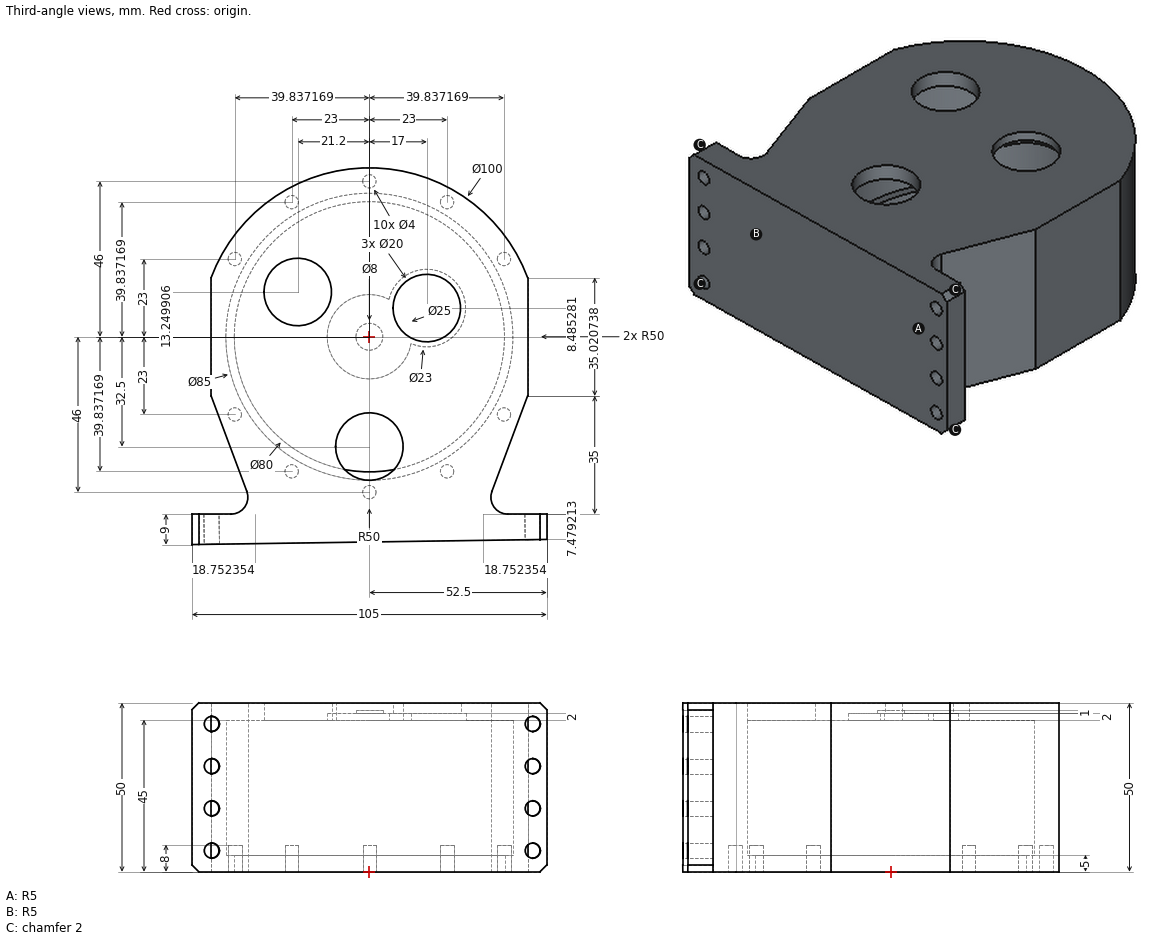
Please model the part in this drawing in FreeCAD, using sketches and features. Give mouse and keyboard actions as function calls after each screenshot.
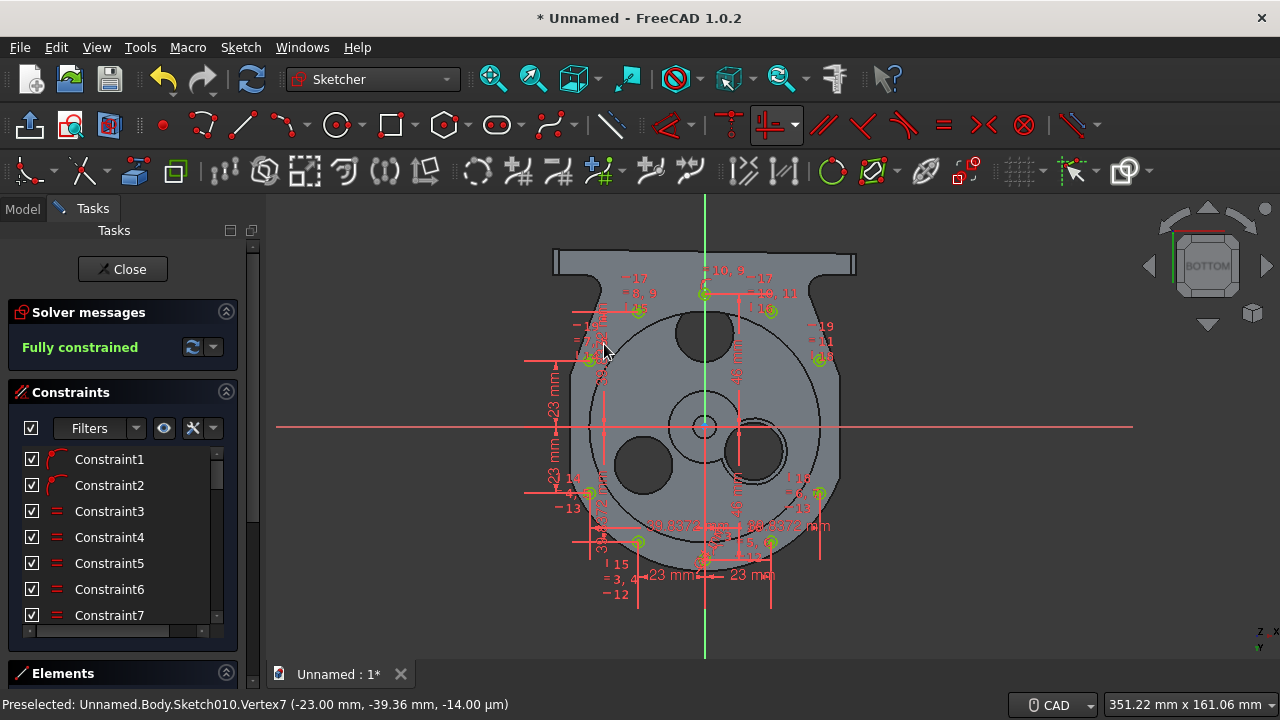
click(123, 269)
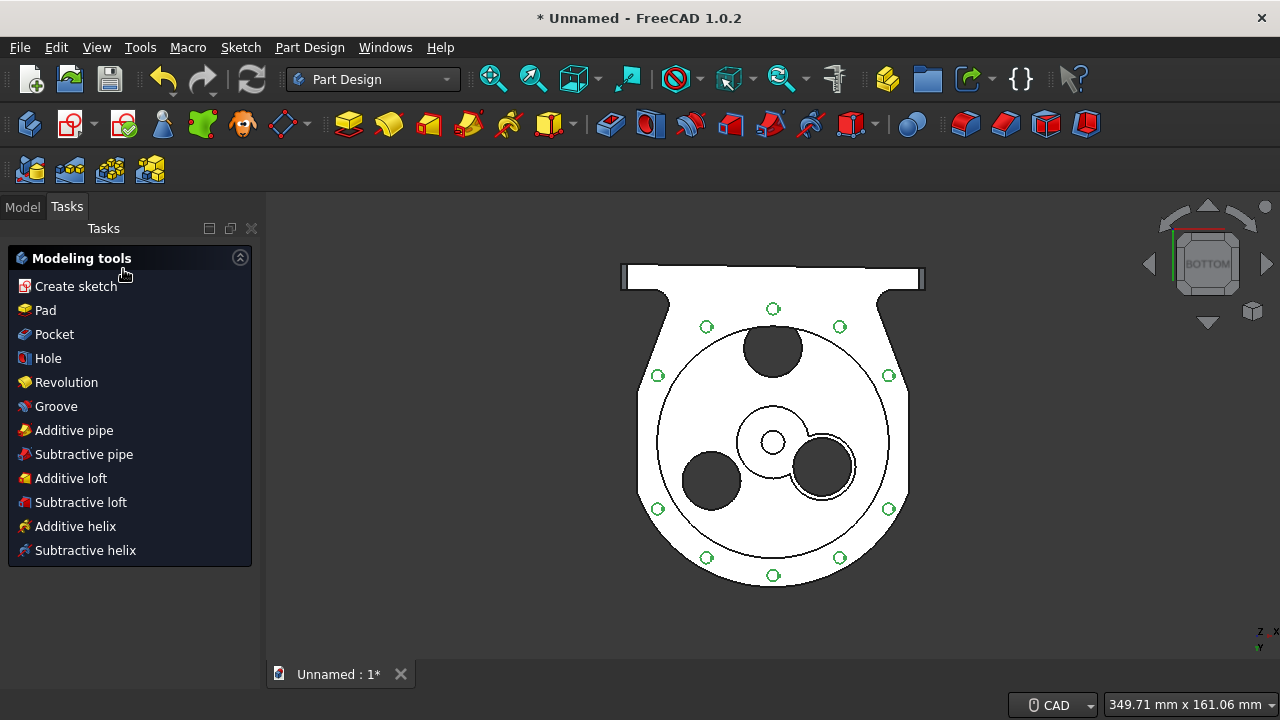
click(612, 124)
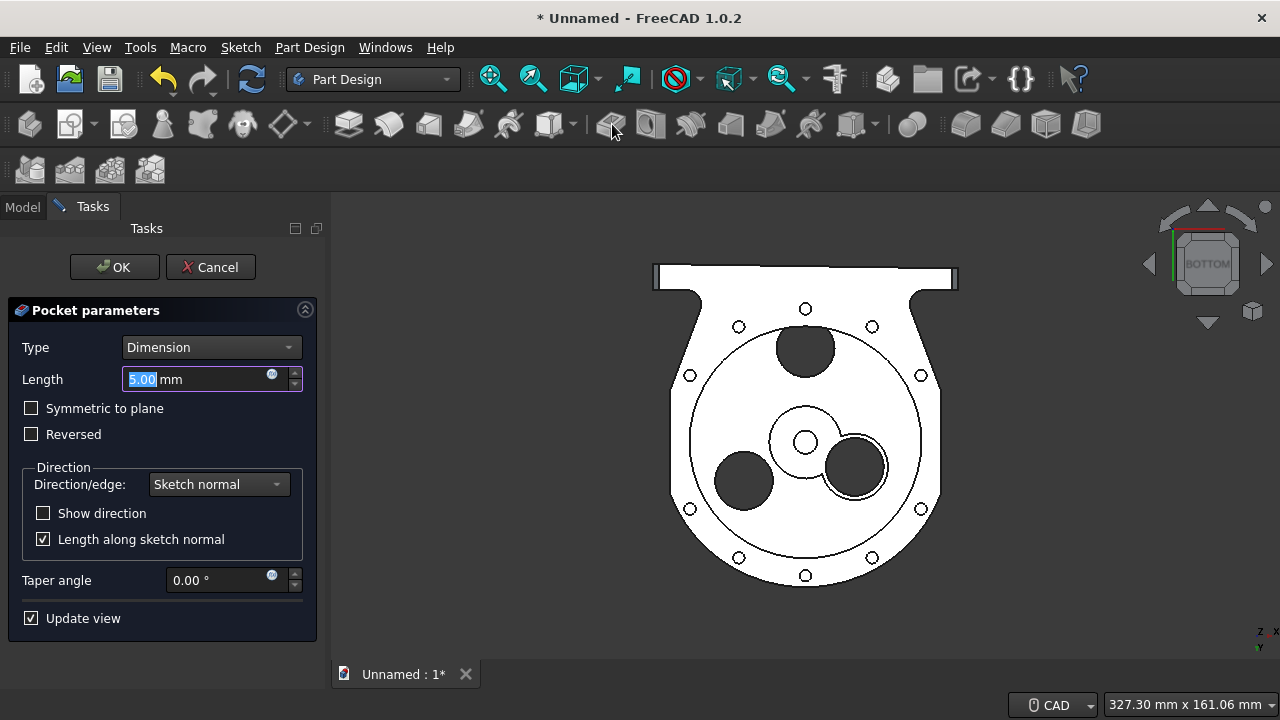
text(8)
key(Tab)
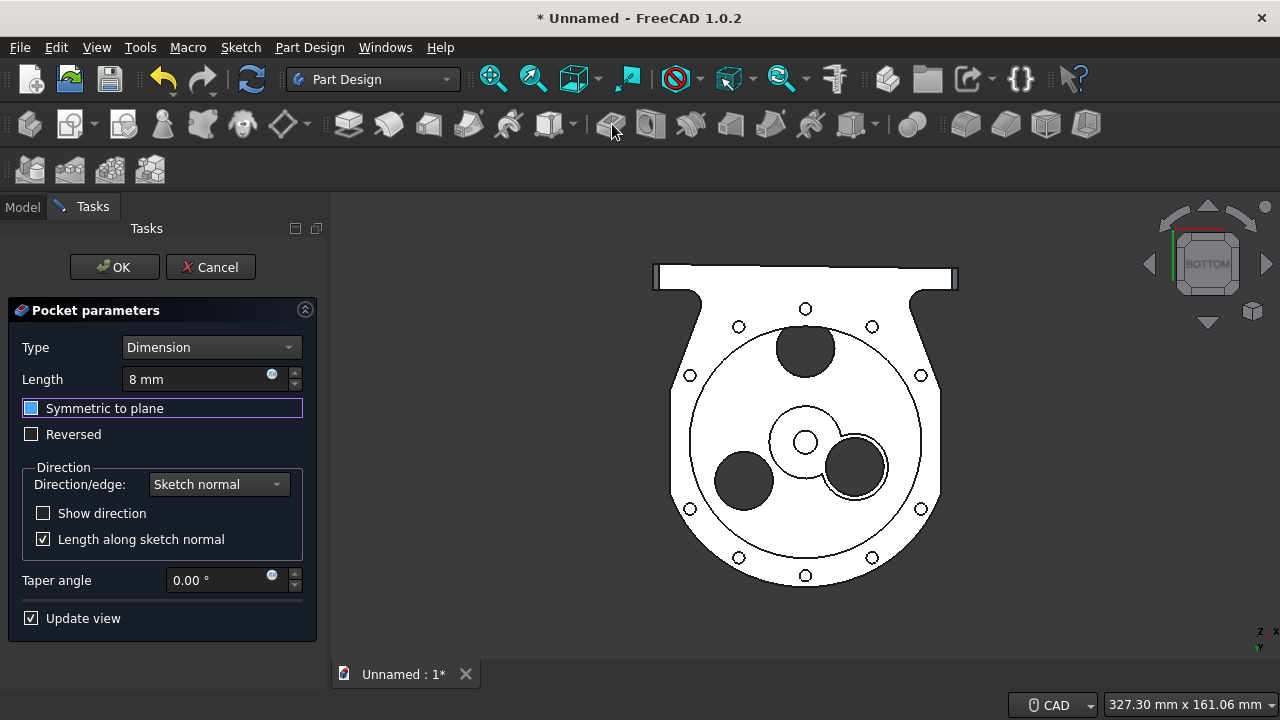
click(115, 267)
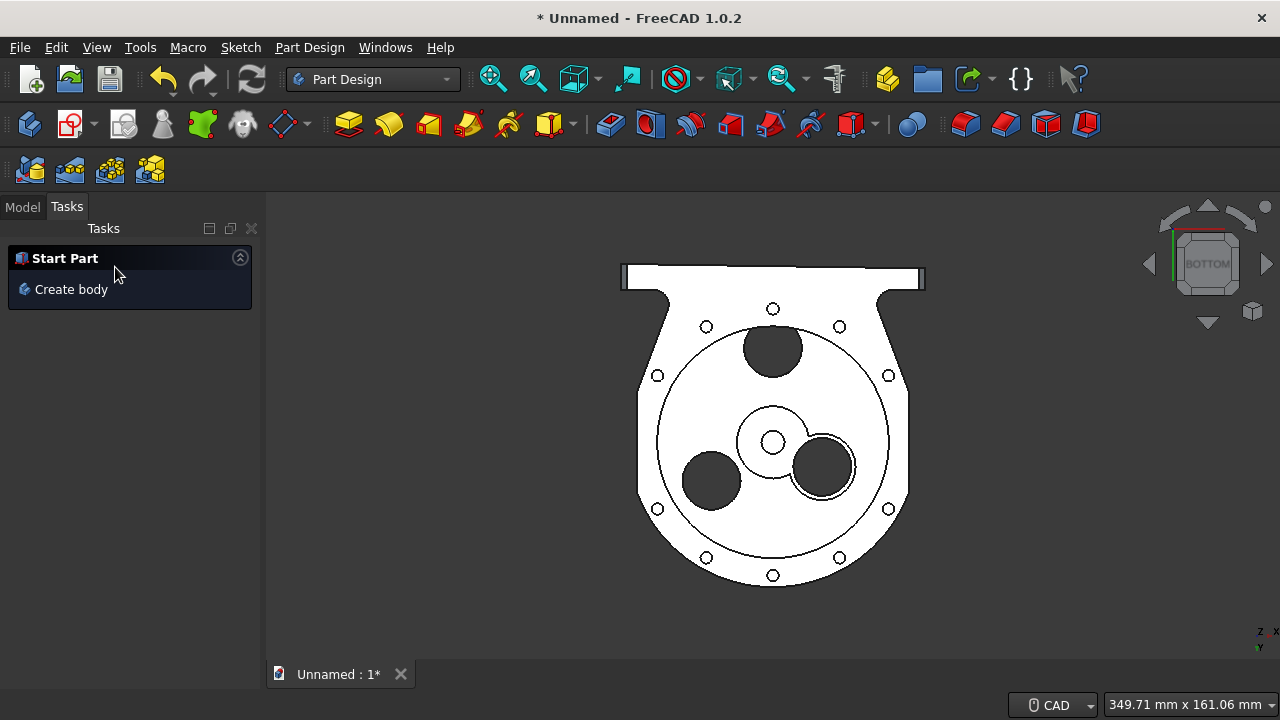
key(0)